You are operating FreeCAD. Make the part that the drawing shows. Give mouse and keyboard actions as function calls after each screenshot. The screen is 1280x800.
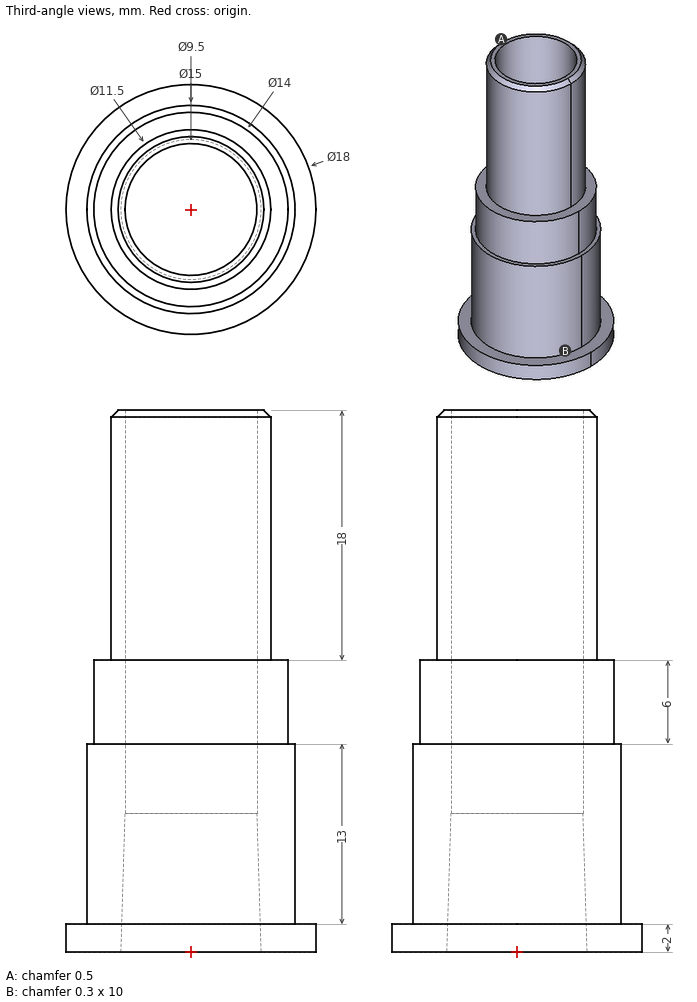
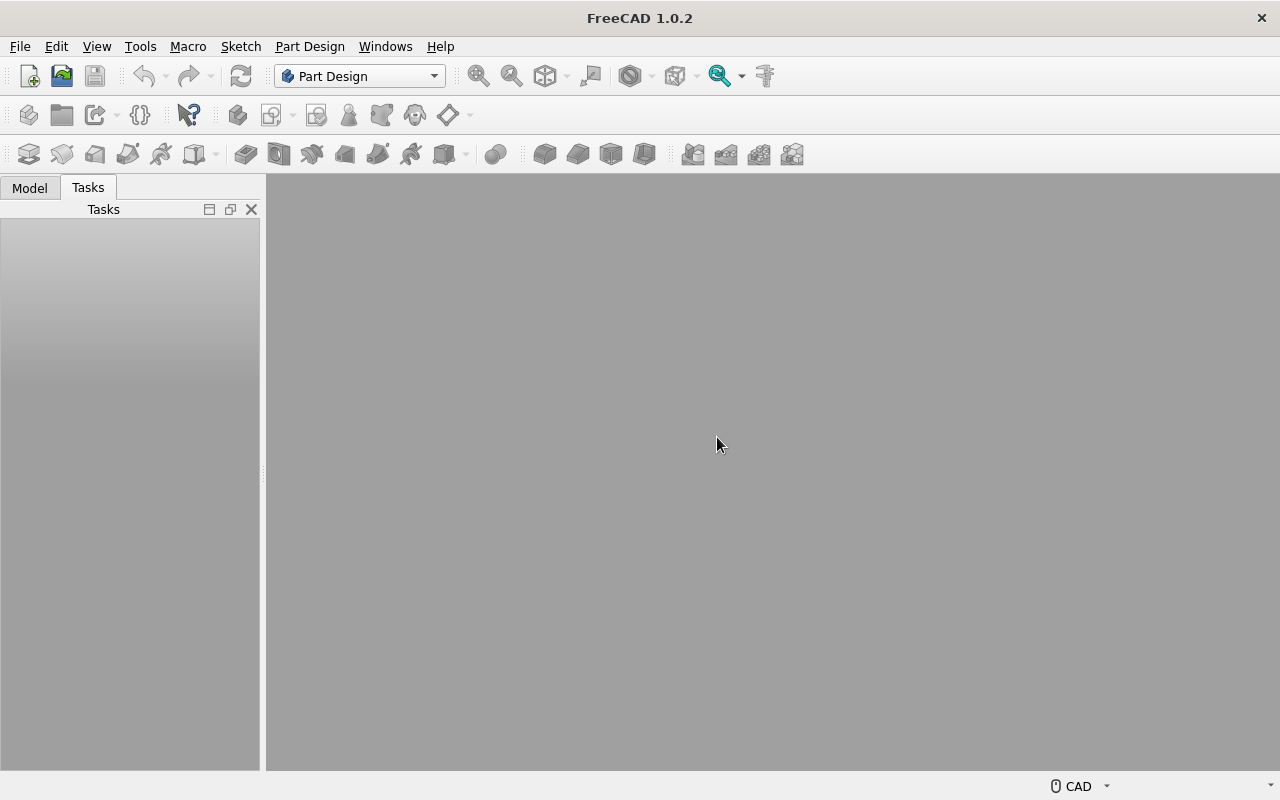
click(29, 76)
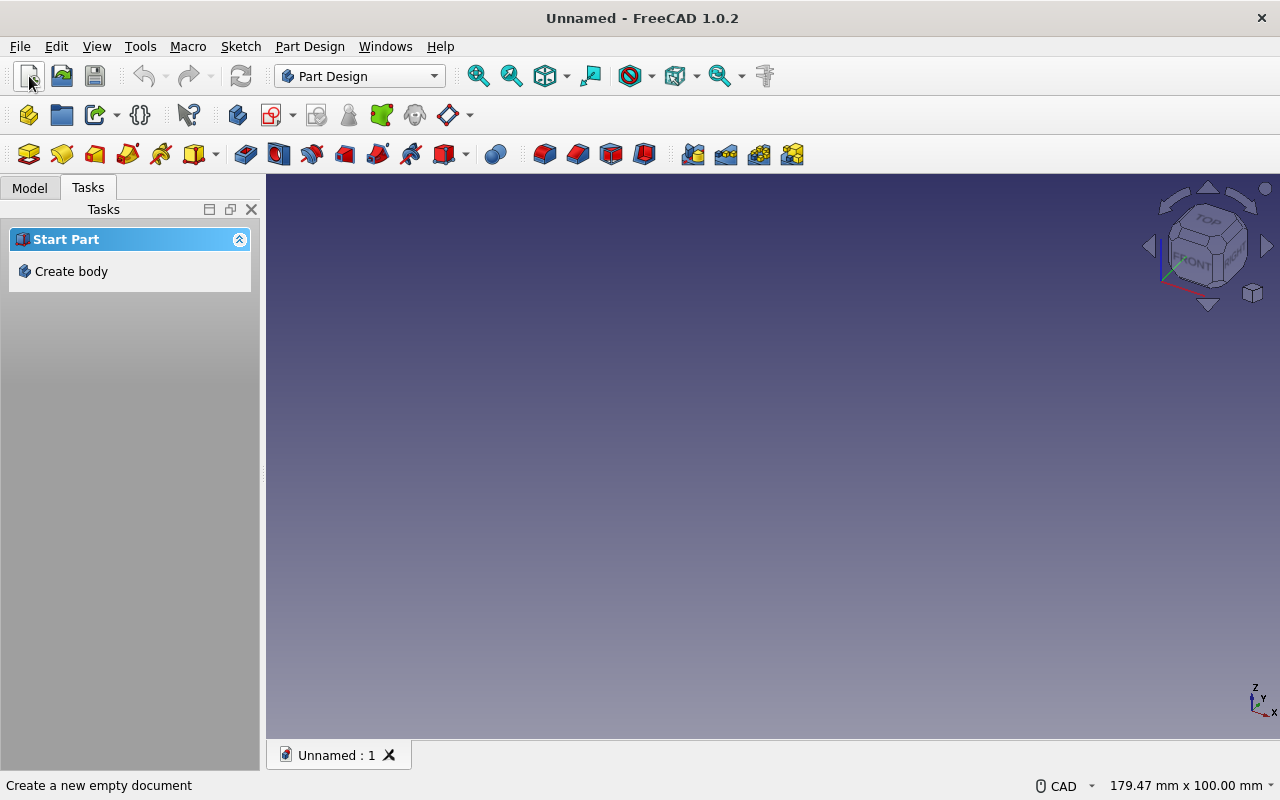
click(270, 116)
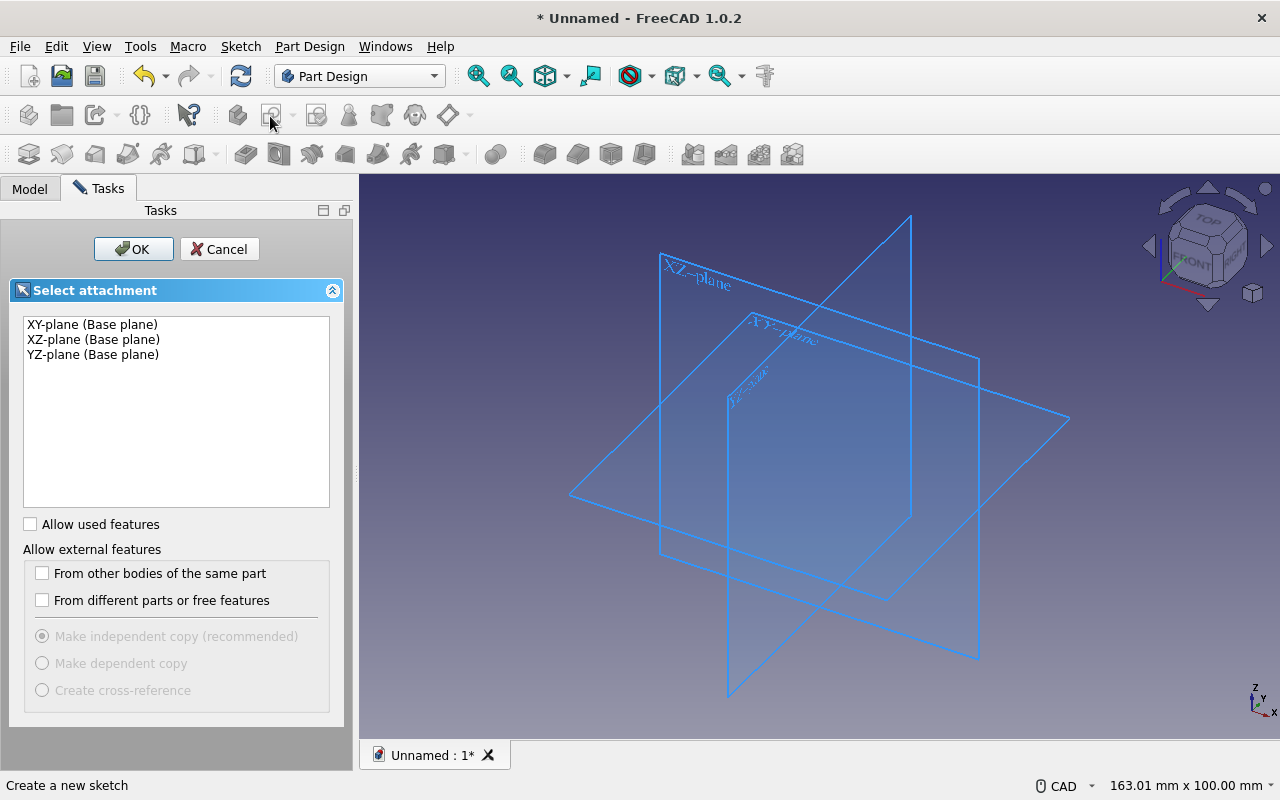
click(84, 324)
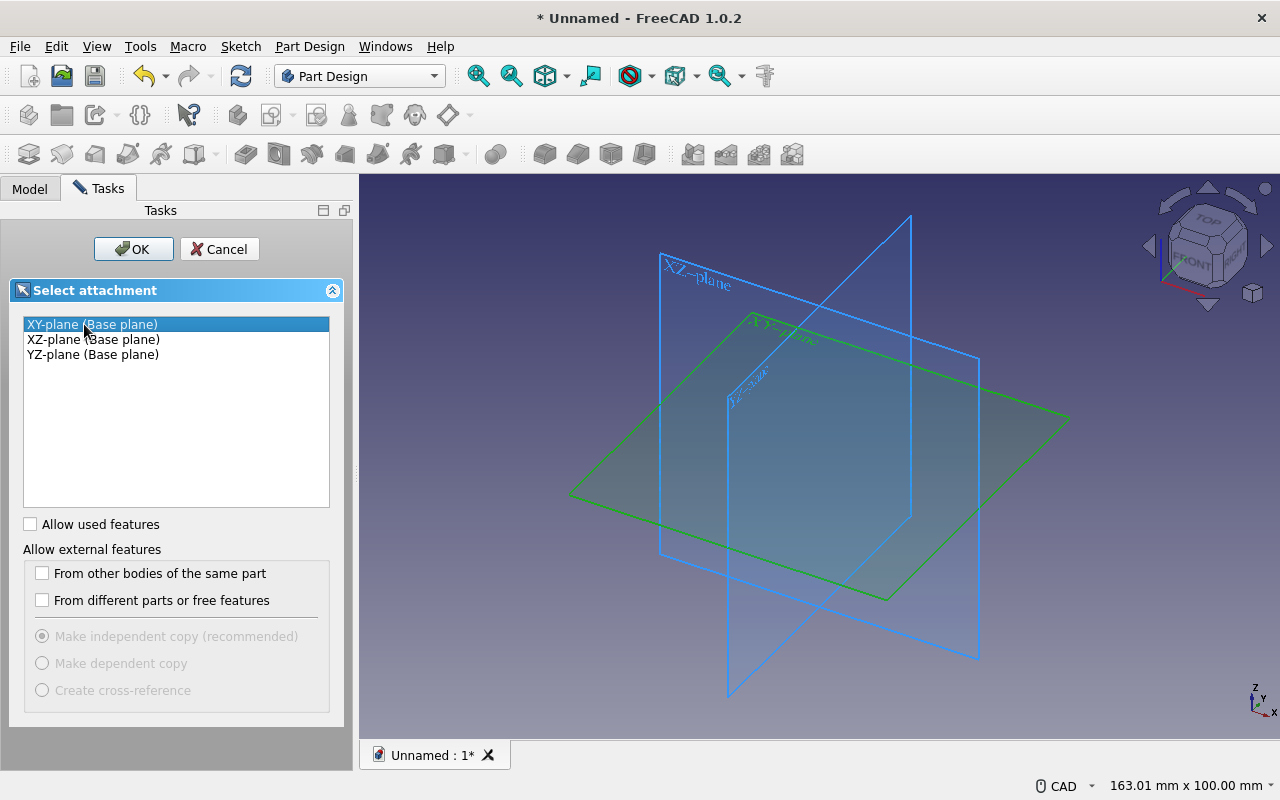
click(134, 249)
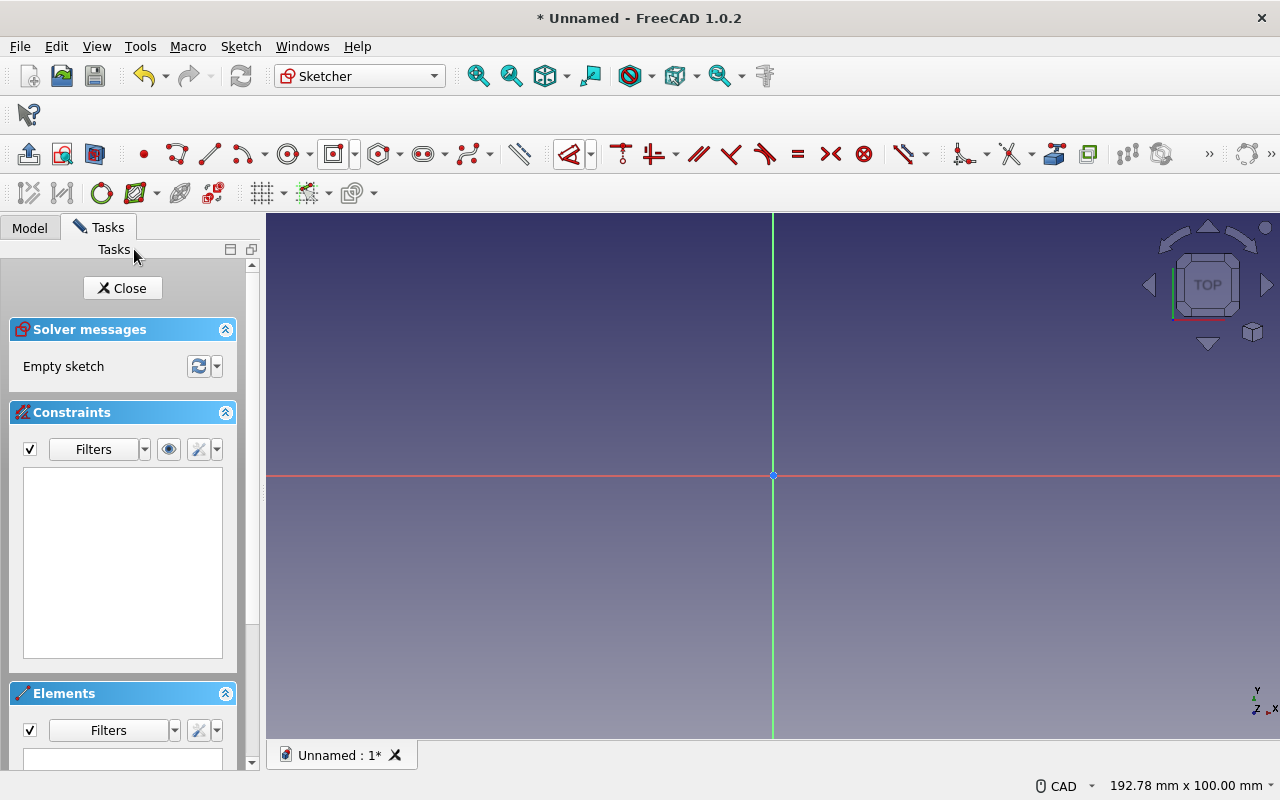
scroll(803, 476, up, 6)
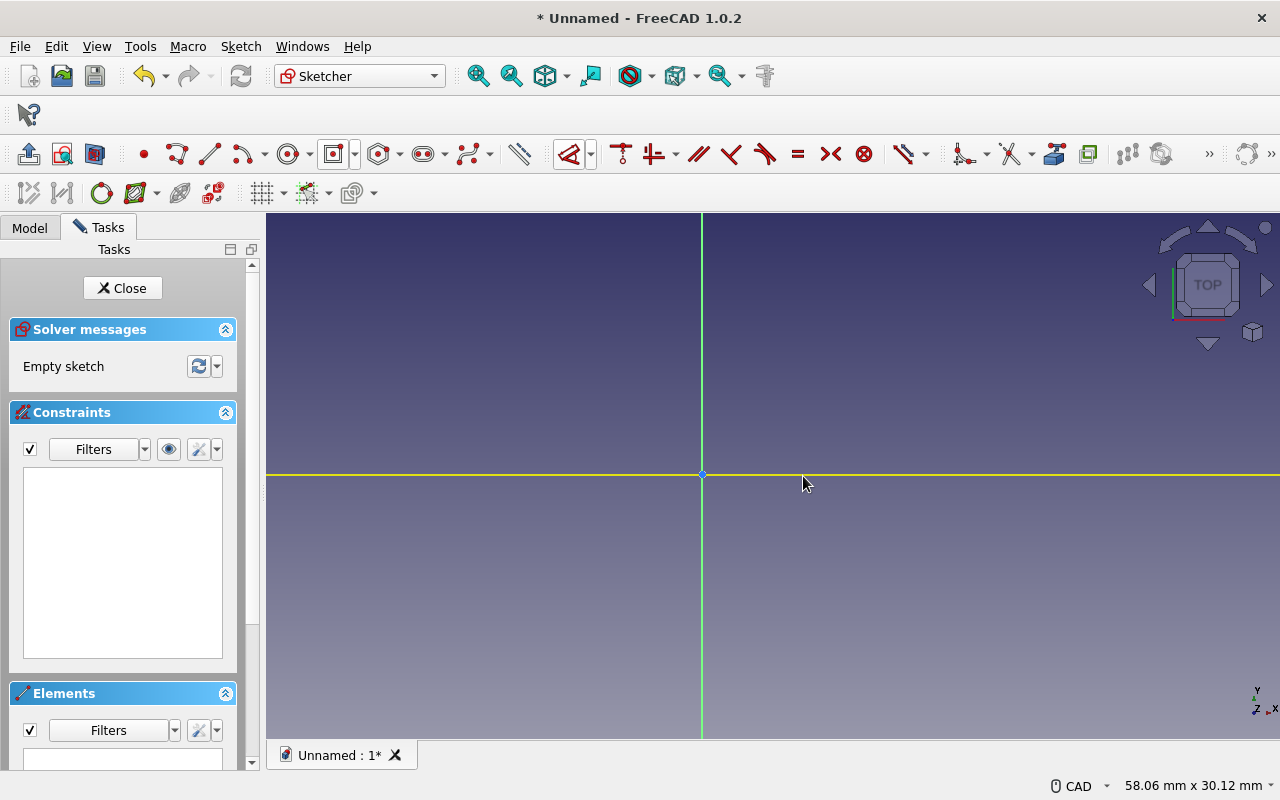
click(288, 154)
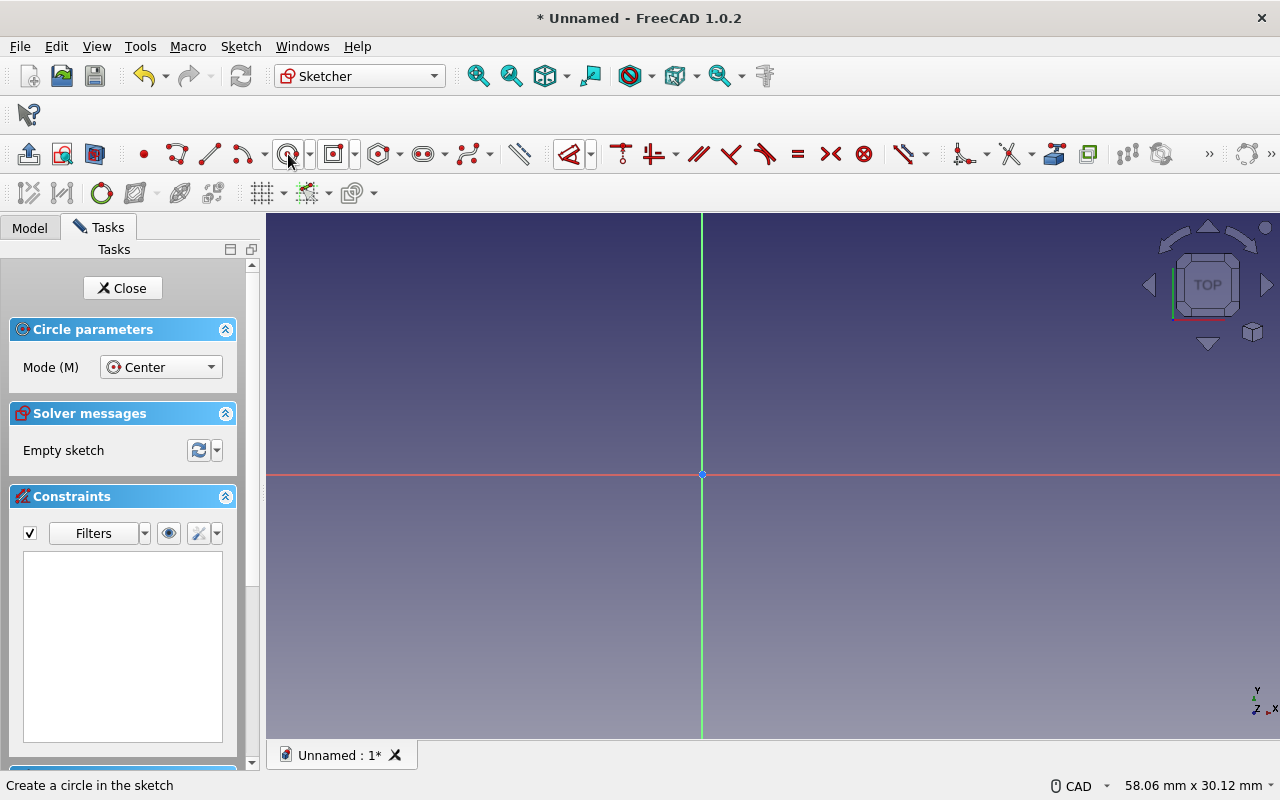
click(702, 475)
click(813, 364)
key(Escape)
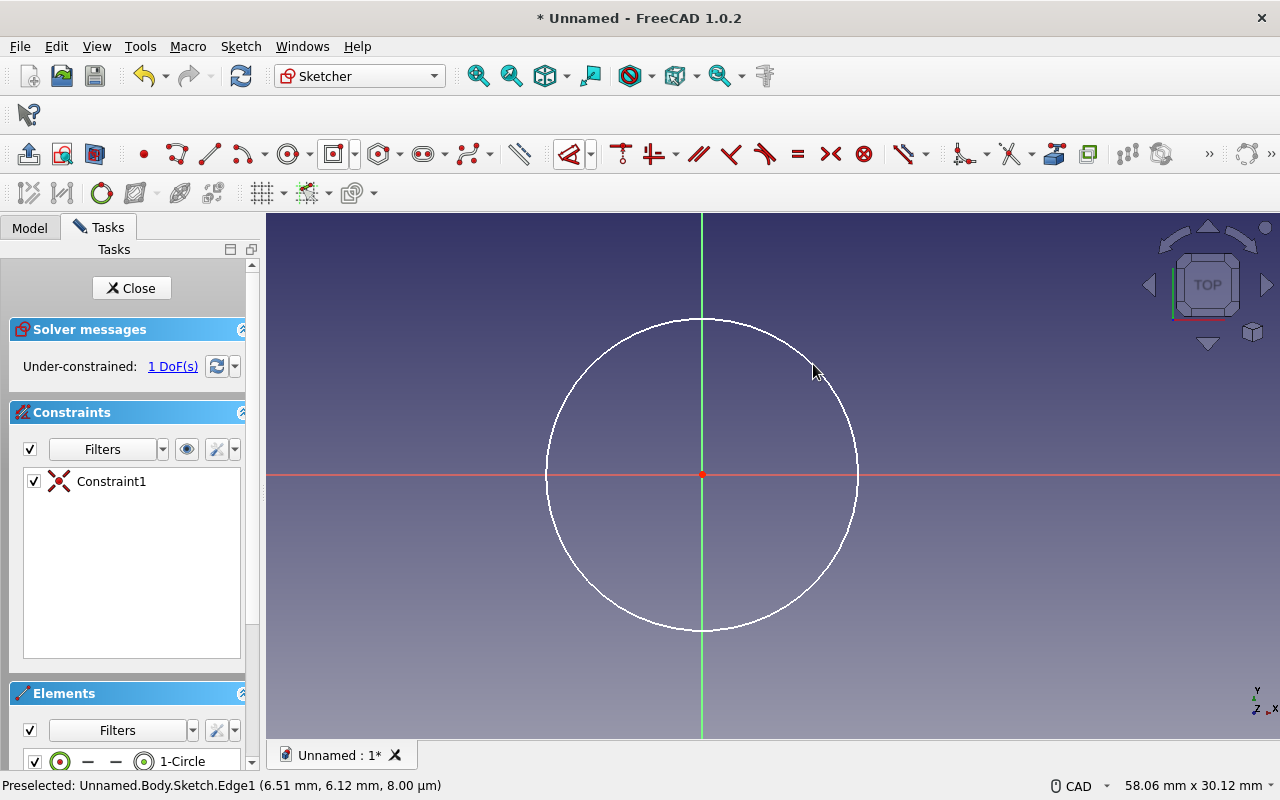
click(568, 154)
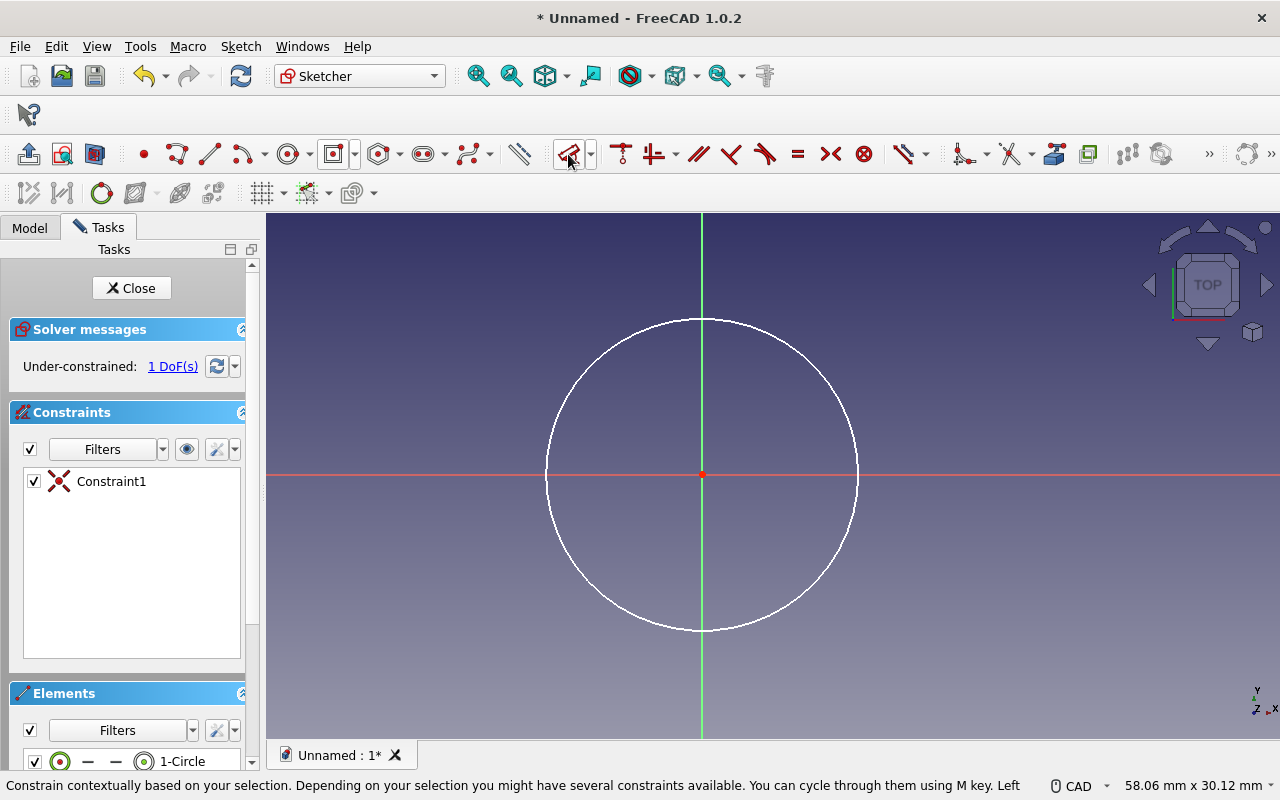
click(812, 364)
click(835, 341)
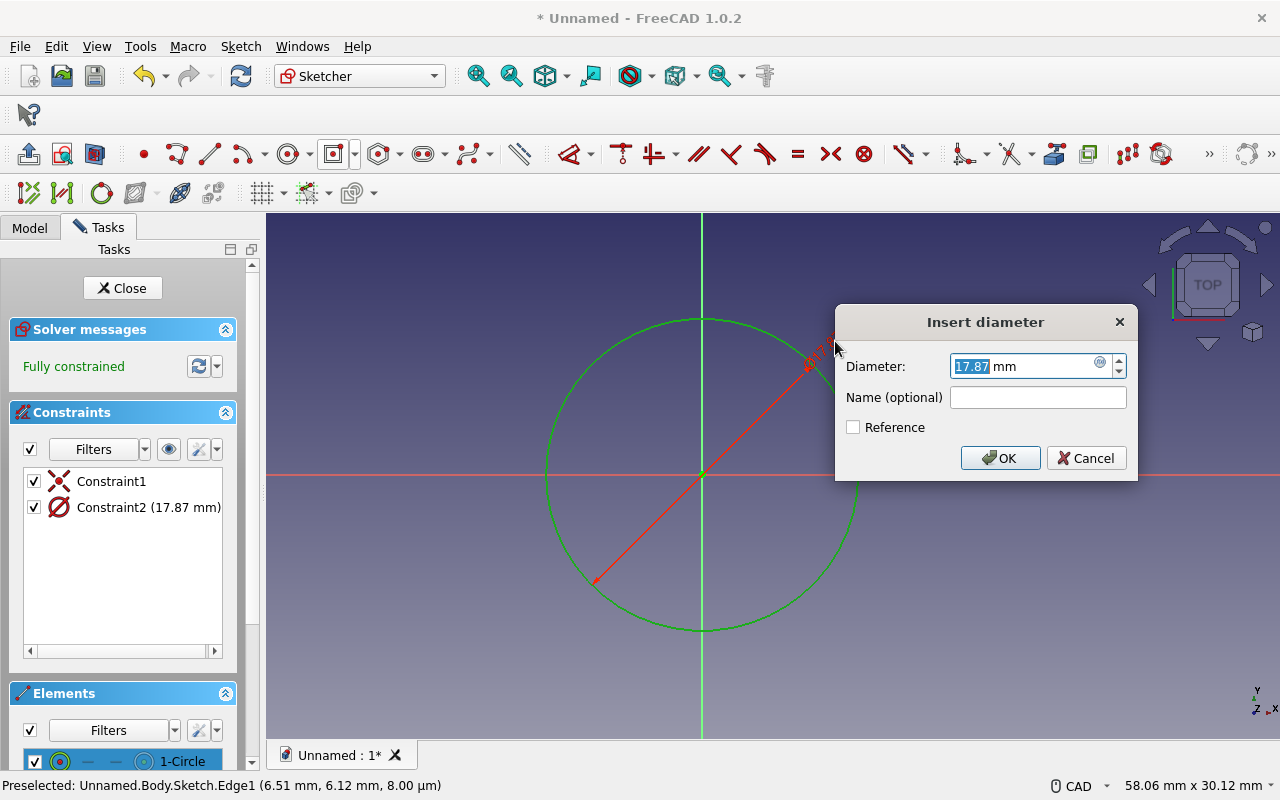
text(18)
key(Return)
key(Escape)